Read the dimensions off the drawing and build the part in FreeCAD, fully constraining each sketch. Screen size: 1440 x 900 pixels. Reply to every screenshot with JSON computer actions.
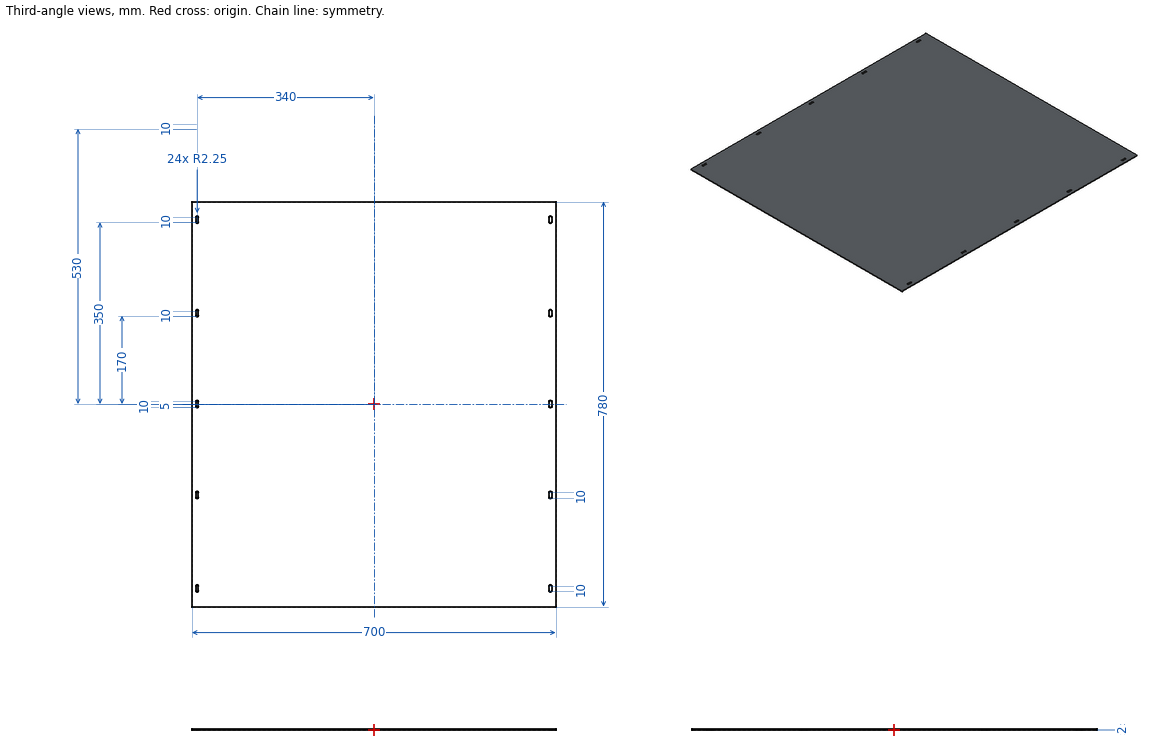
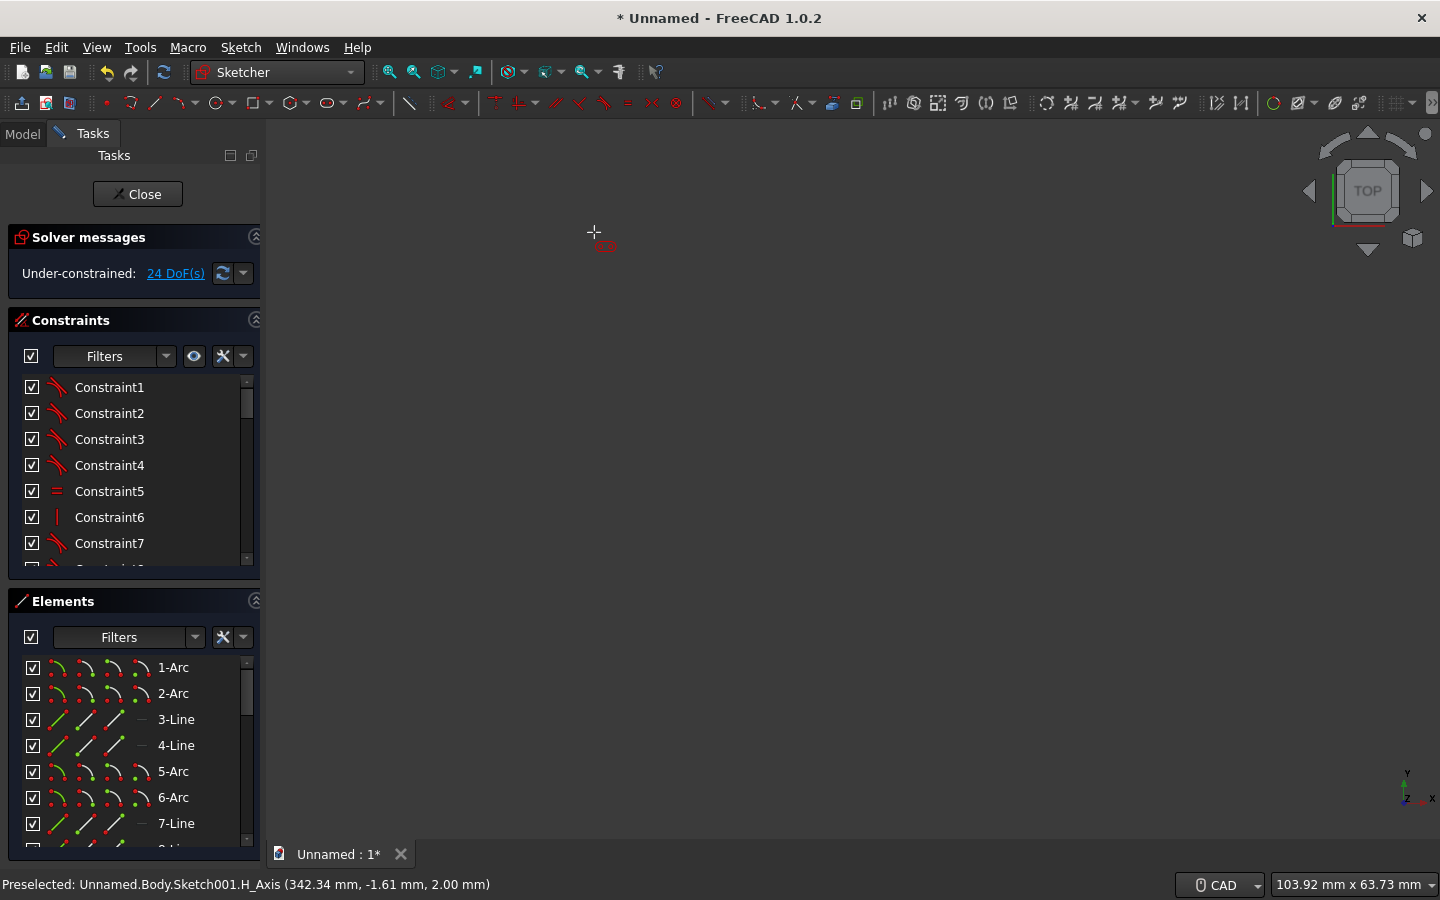
{"action": "scroll", "coordinate": [594, 232], "scroll_direction": "down", "scroll_amount": 15}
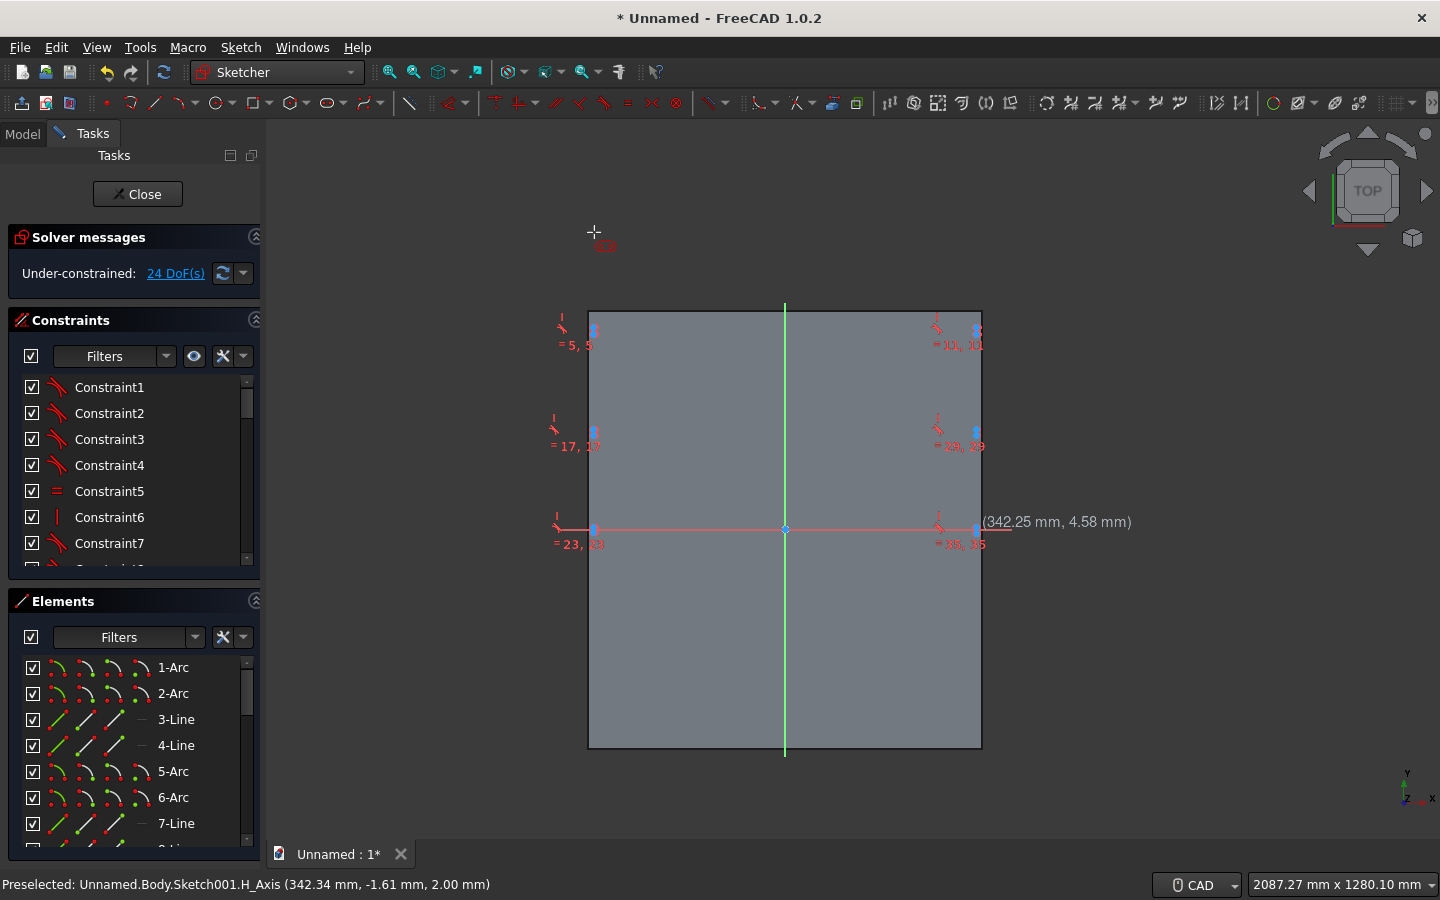
{"action": "left_click", "coordinate": [594, 232]}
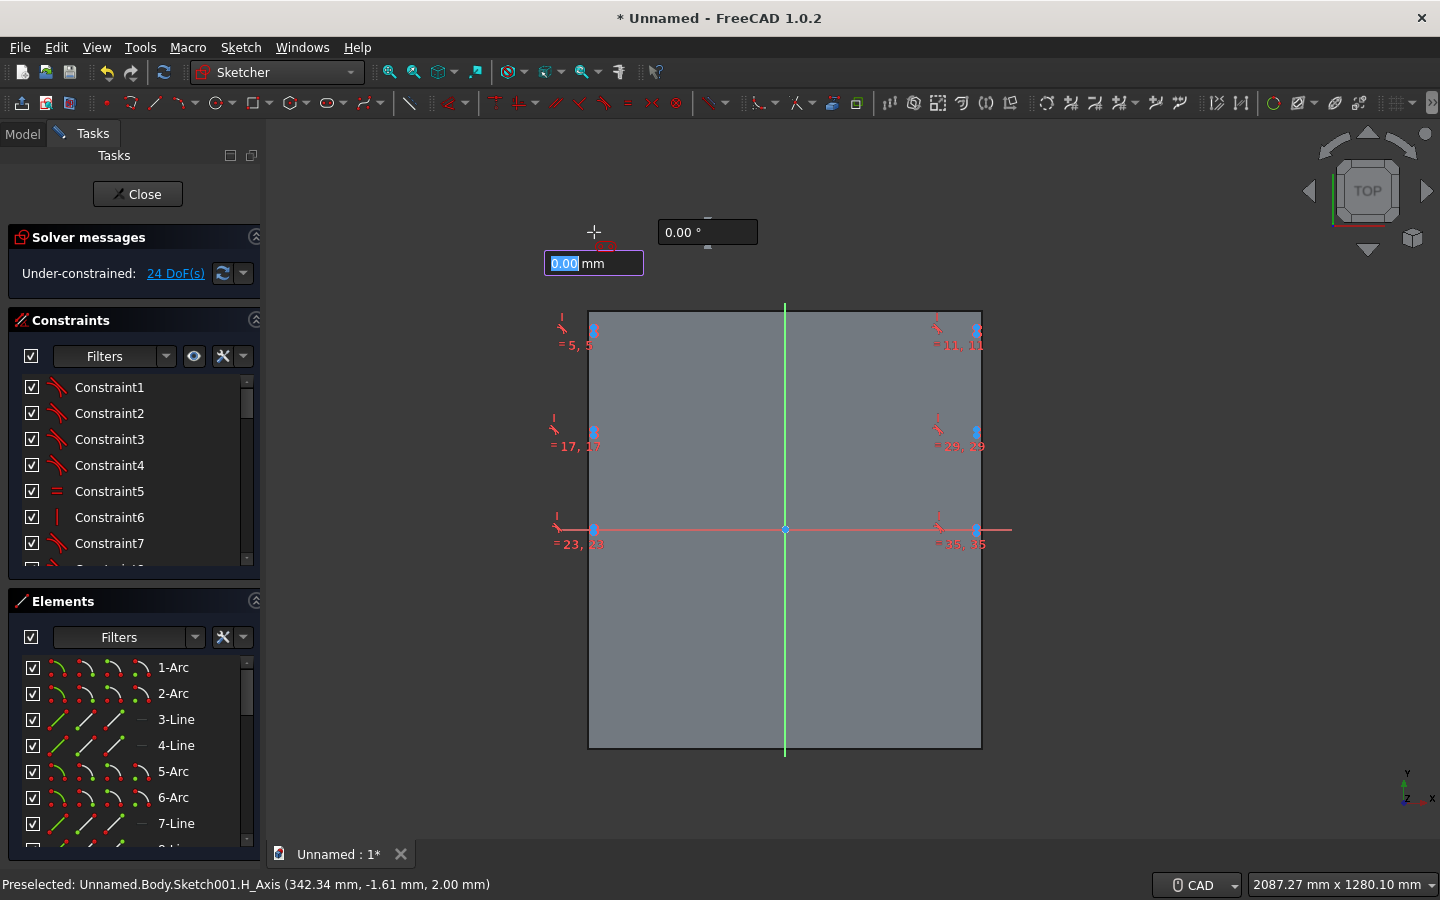
{"action": "scroll", "coordinate": [594, 226], "scroll_direction": "up", "scroll_amount": 6}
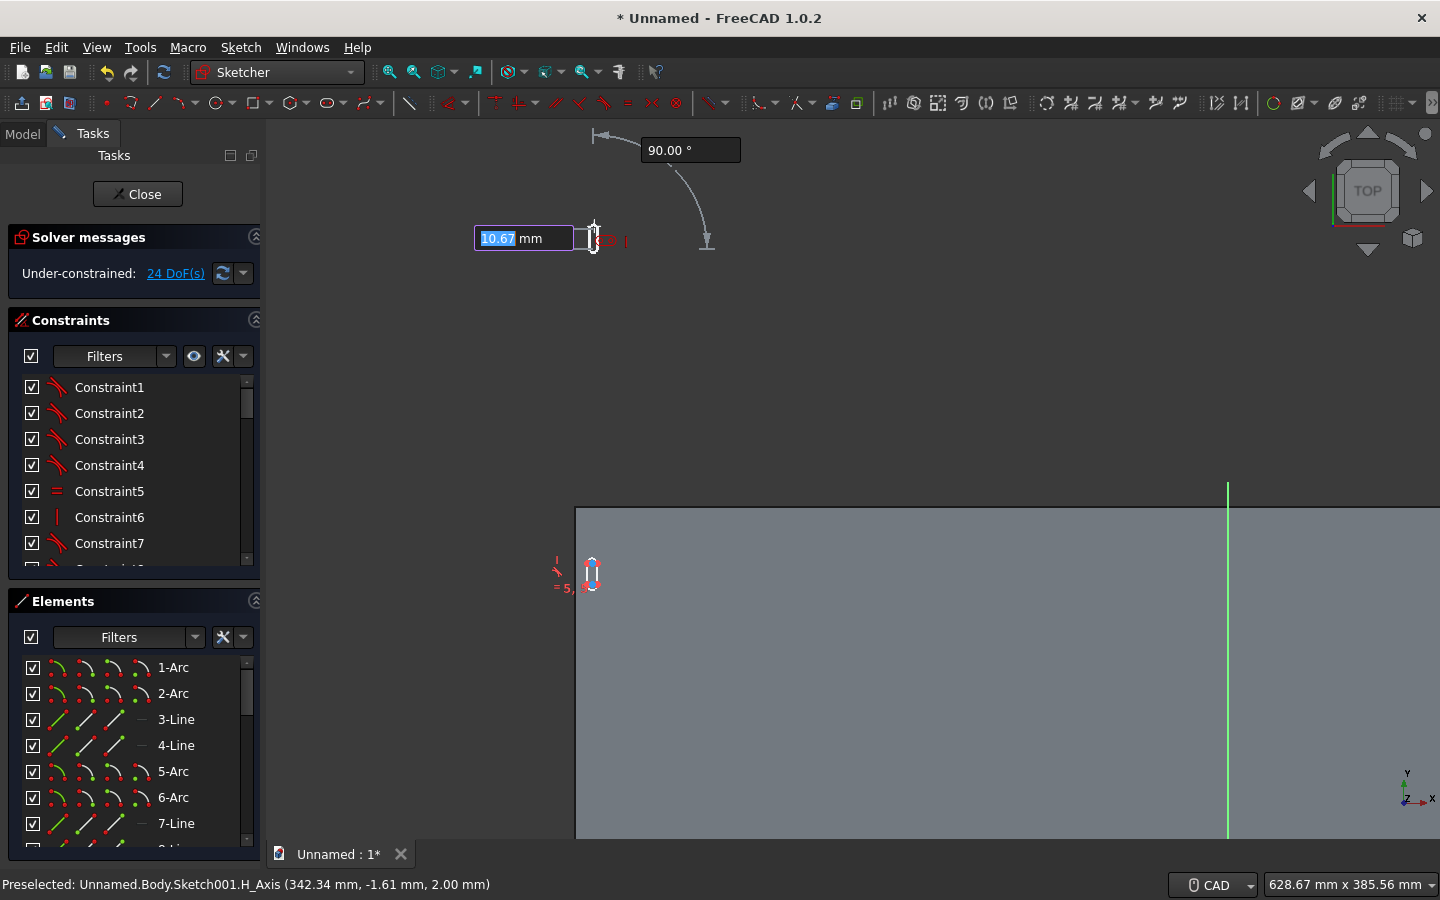
{"action": "left_click", "coordinate": [593, 227]}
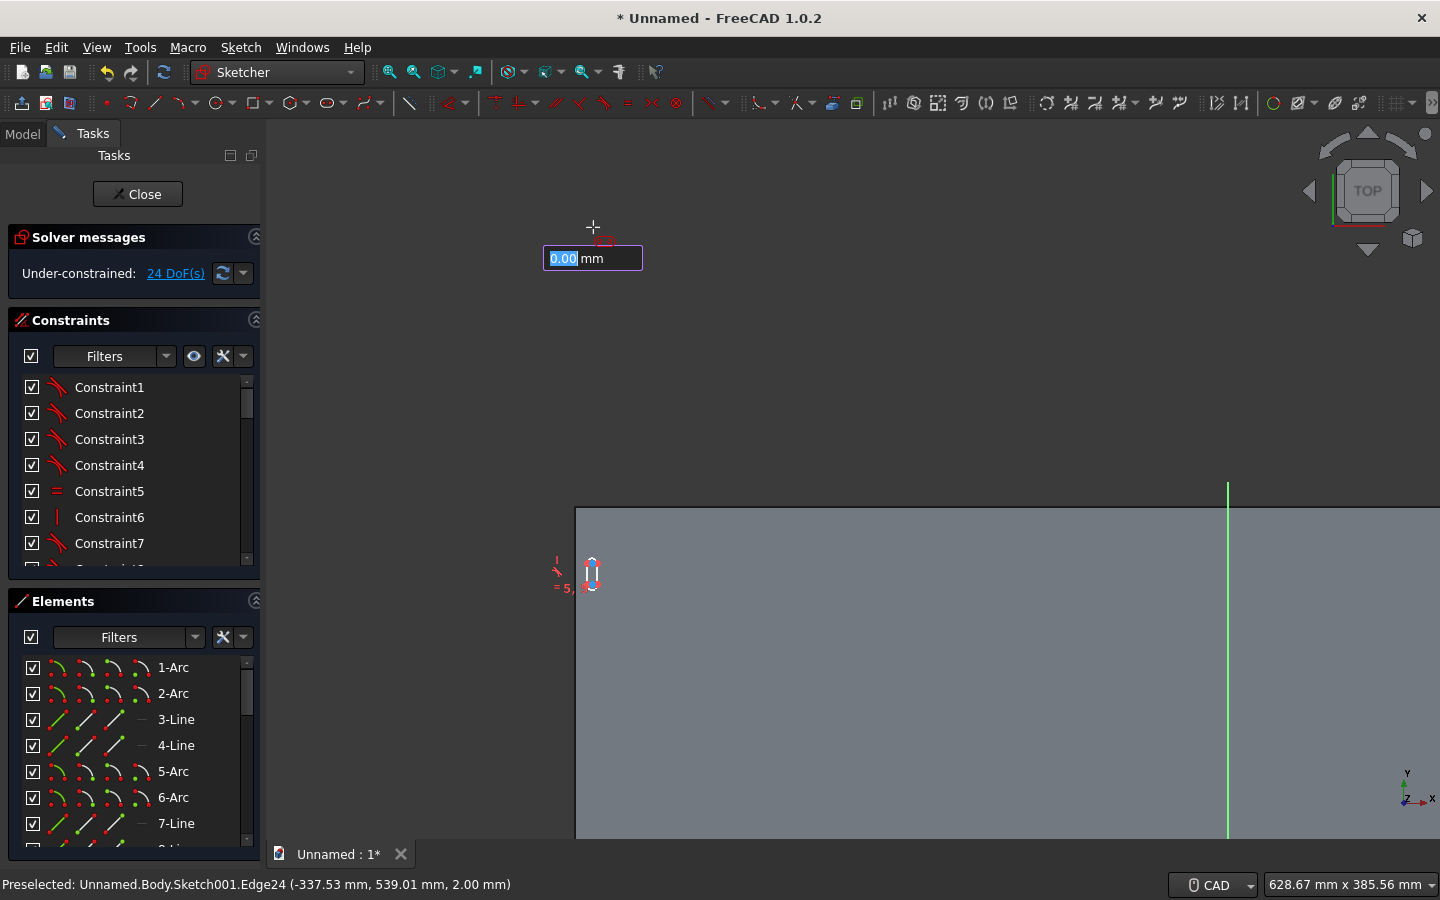
{"action": "scroll", "coordinate": [589, 236], "scroll_direction": "up", "scroll_amount": 7}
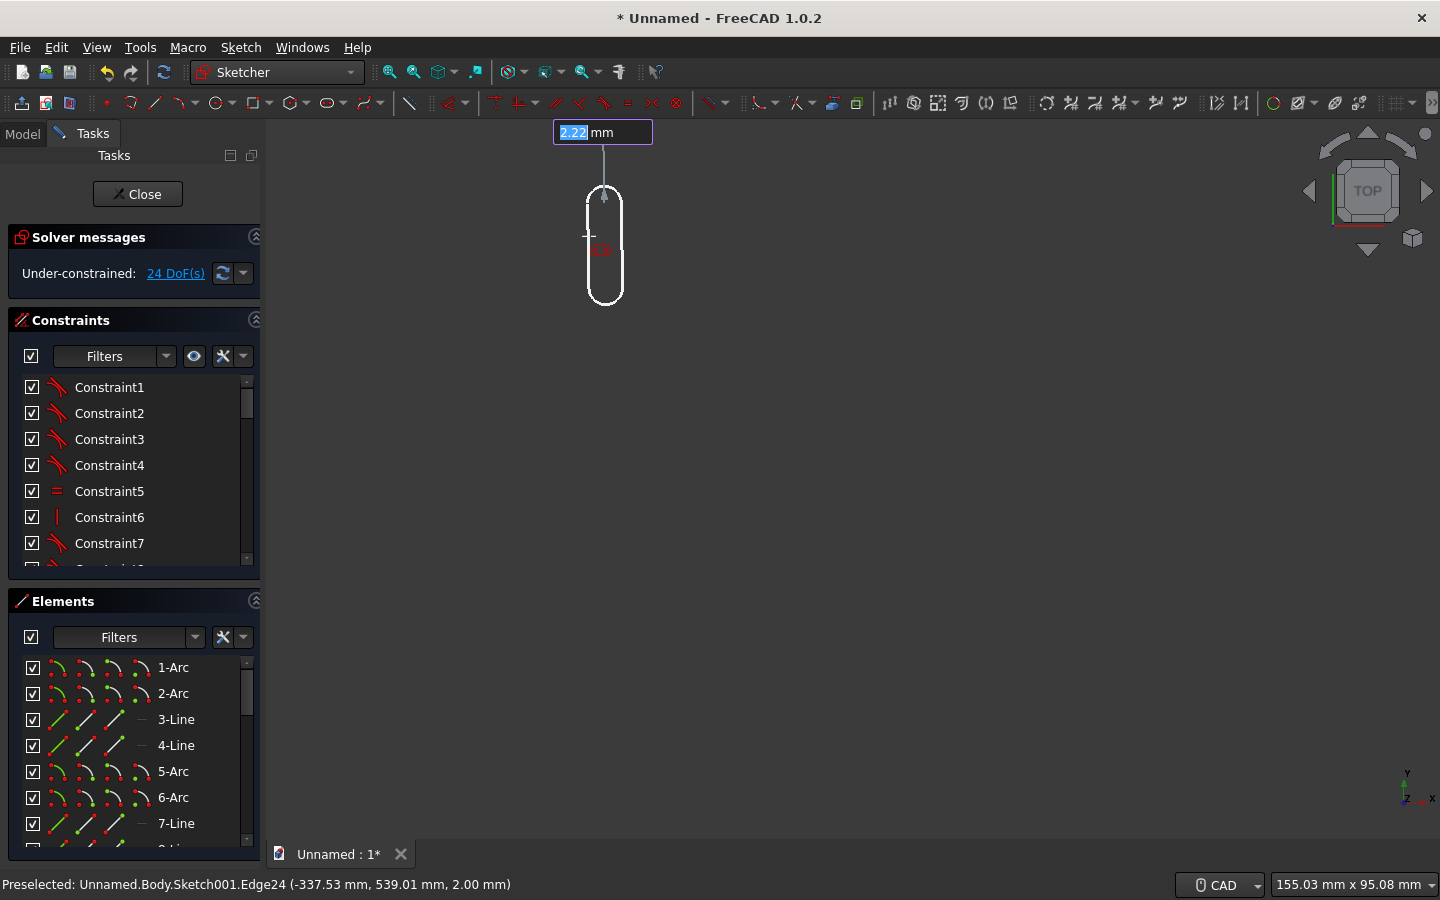
{"action": "left_click", "coordinate": [589, 235]}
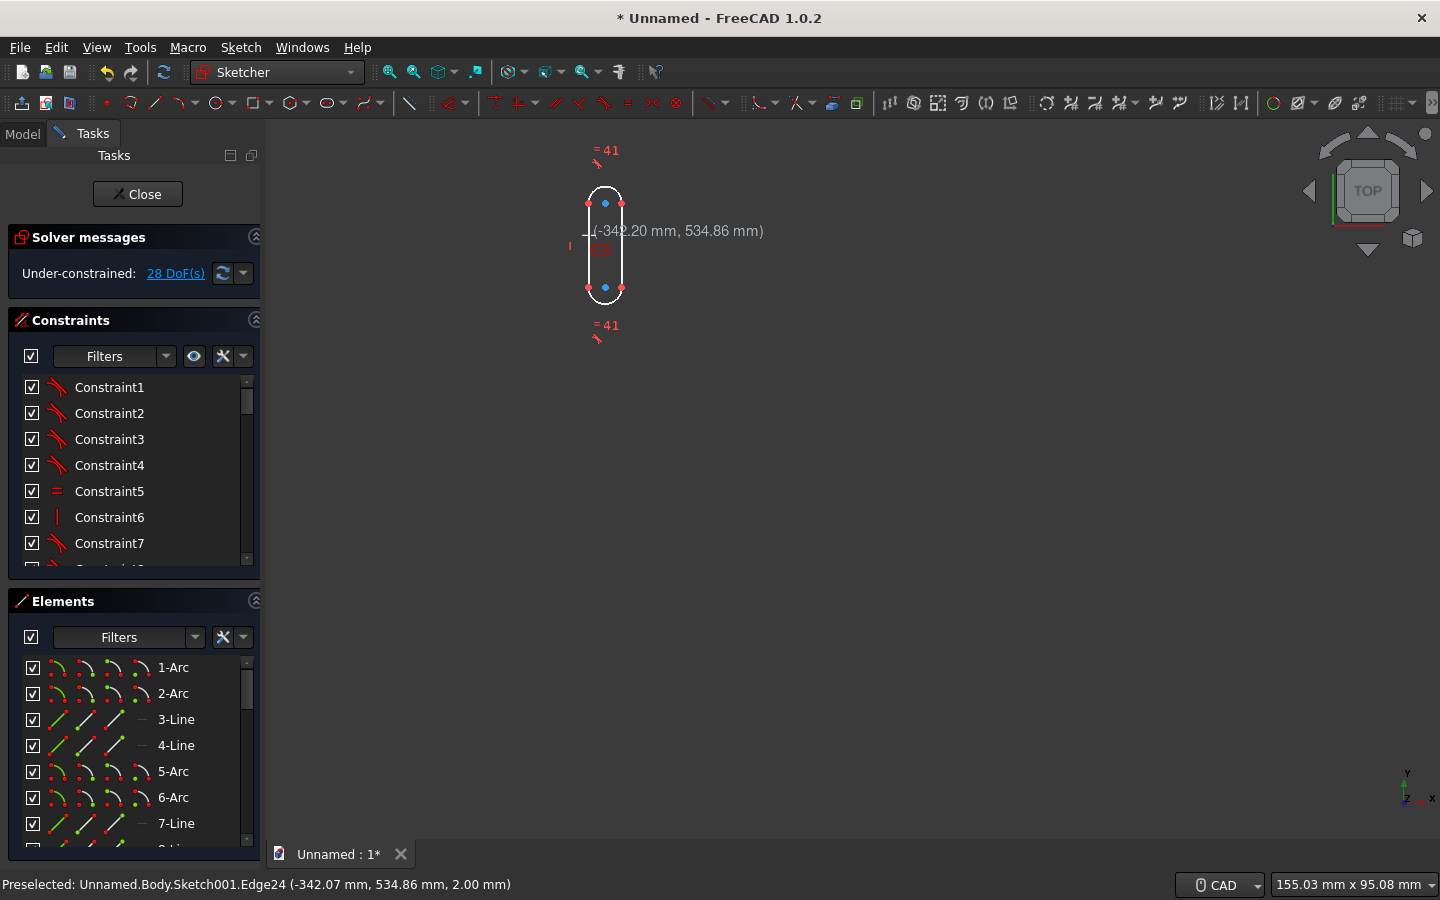
{"action": "scroll", "coordinate": [592, 228], "scroll_direction": "down", "scroll_amount": 13}